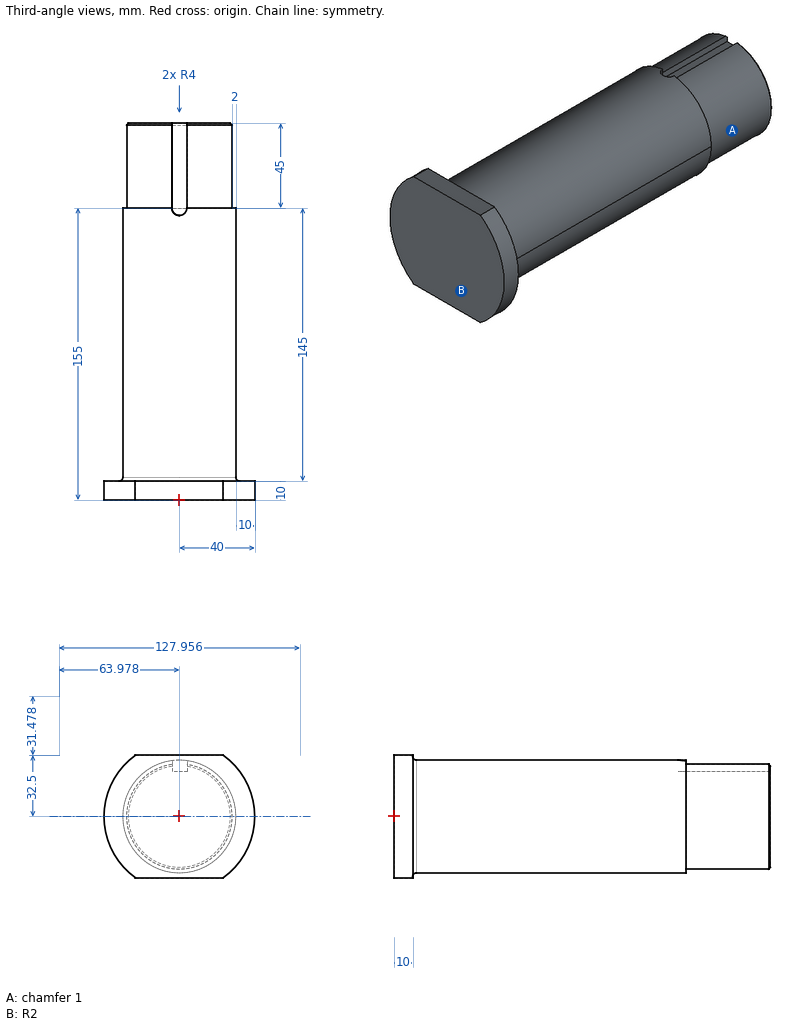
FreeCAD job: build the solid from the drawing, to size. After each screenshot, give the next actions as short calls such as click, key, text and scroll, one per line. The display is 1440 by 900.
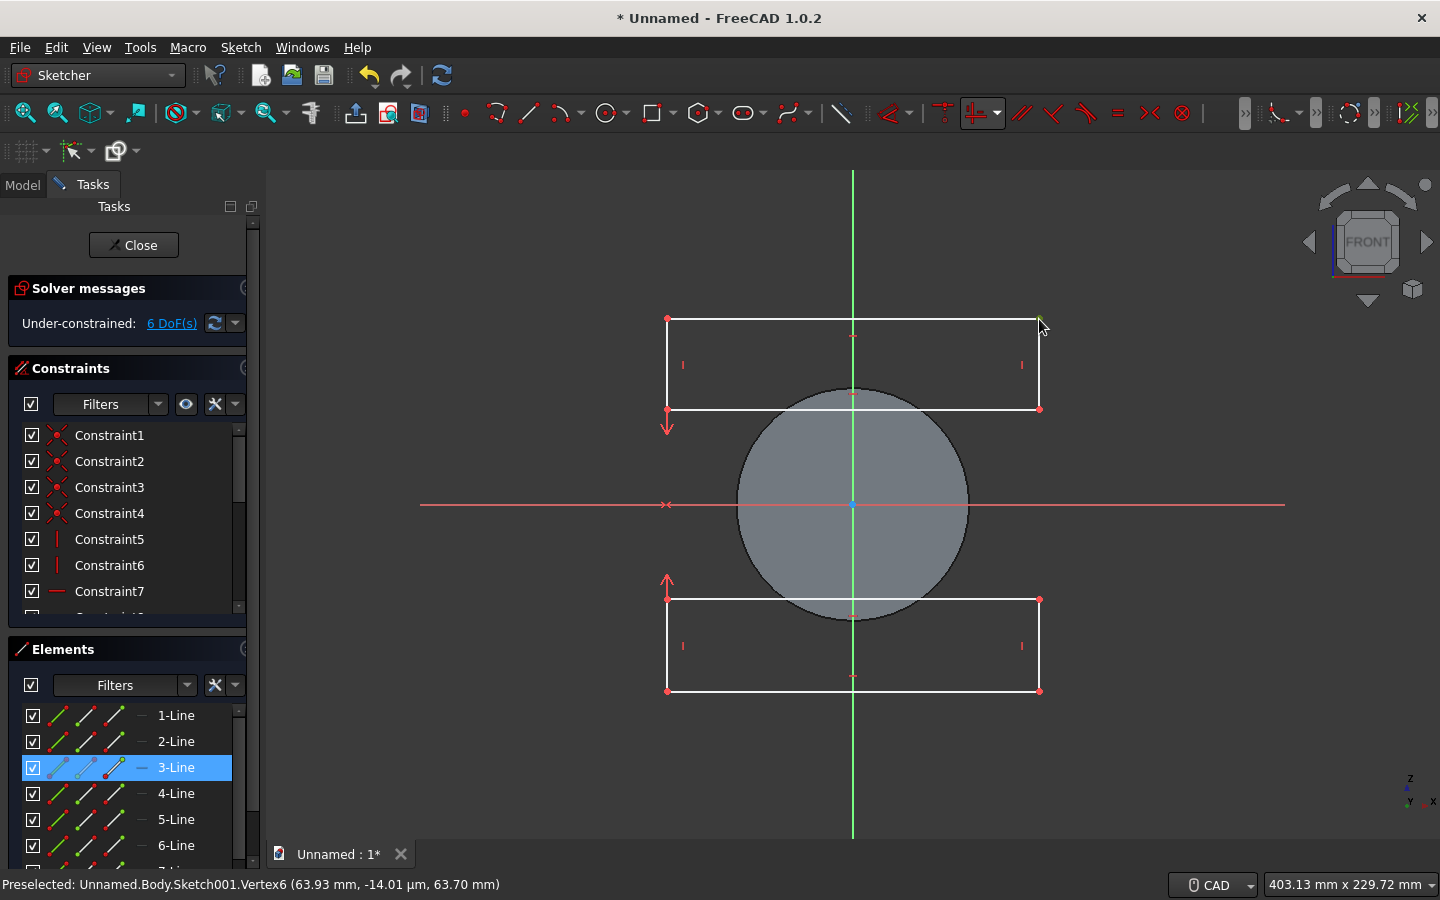
click(1039, 692)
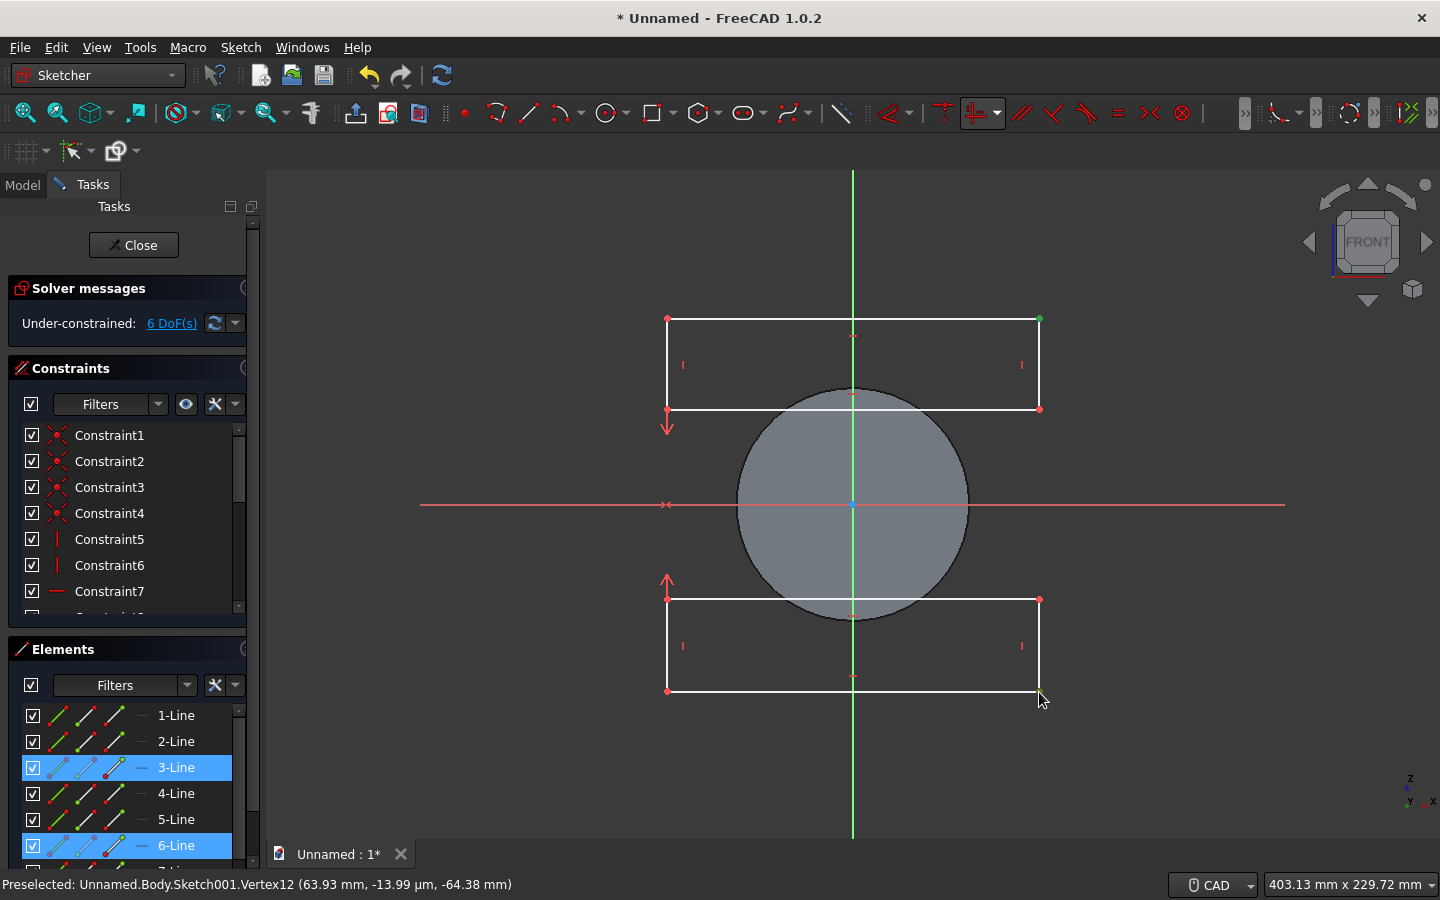
click(434, 505)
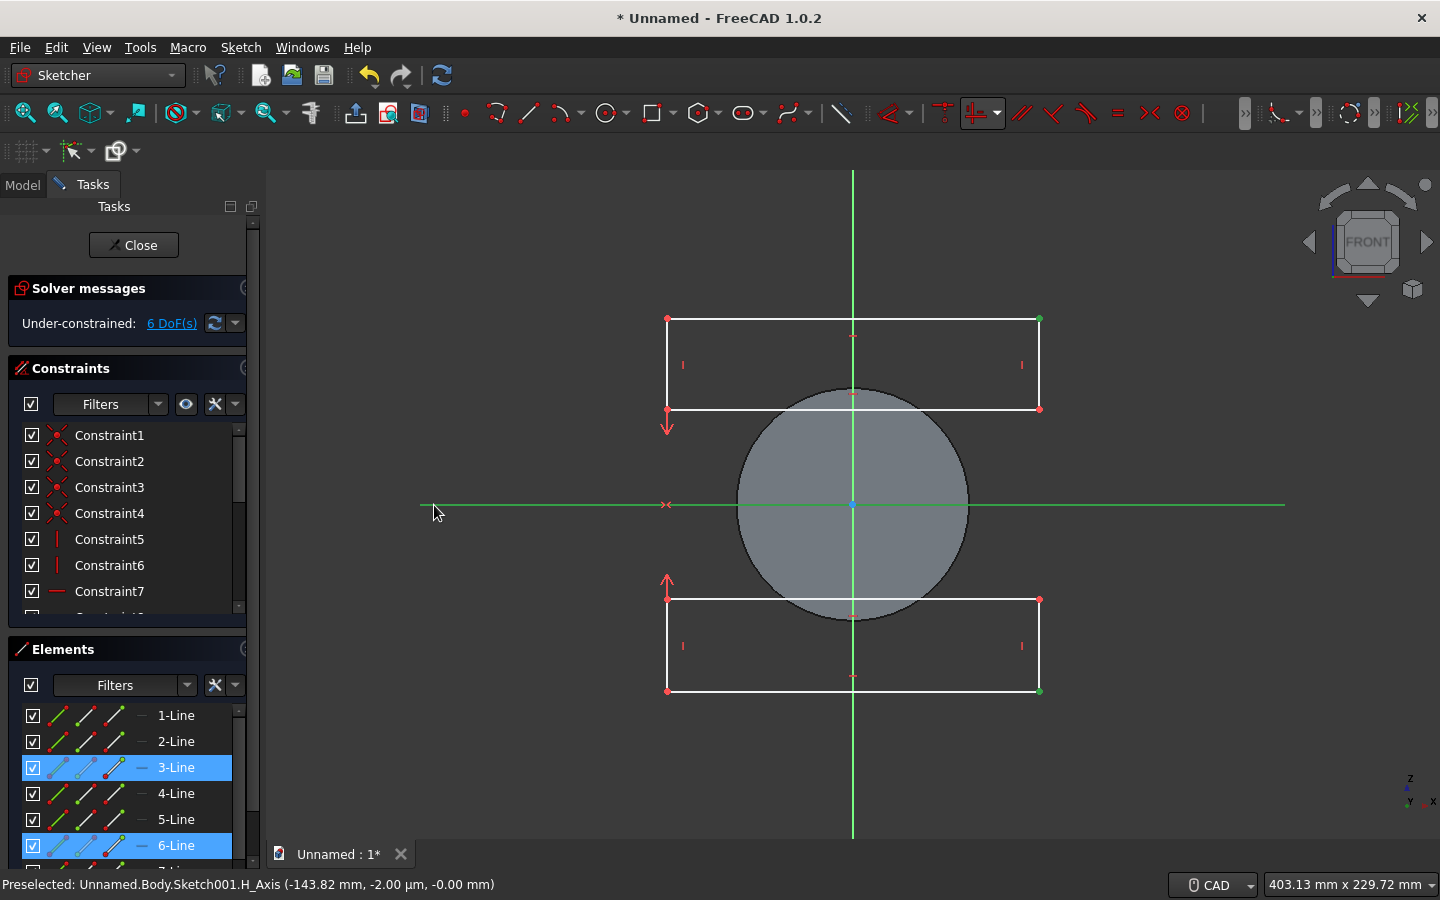
click(1150, 114)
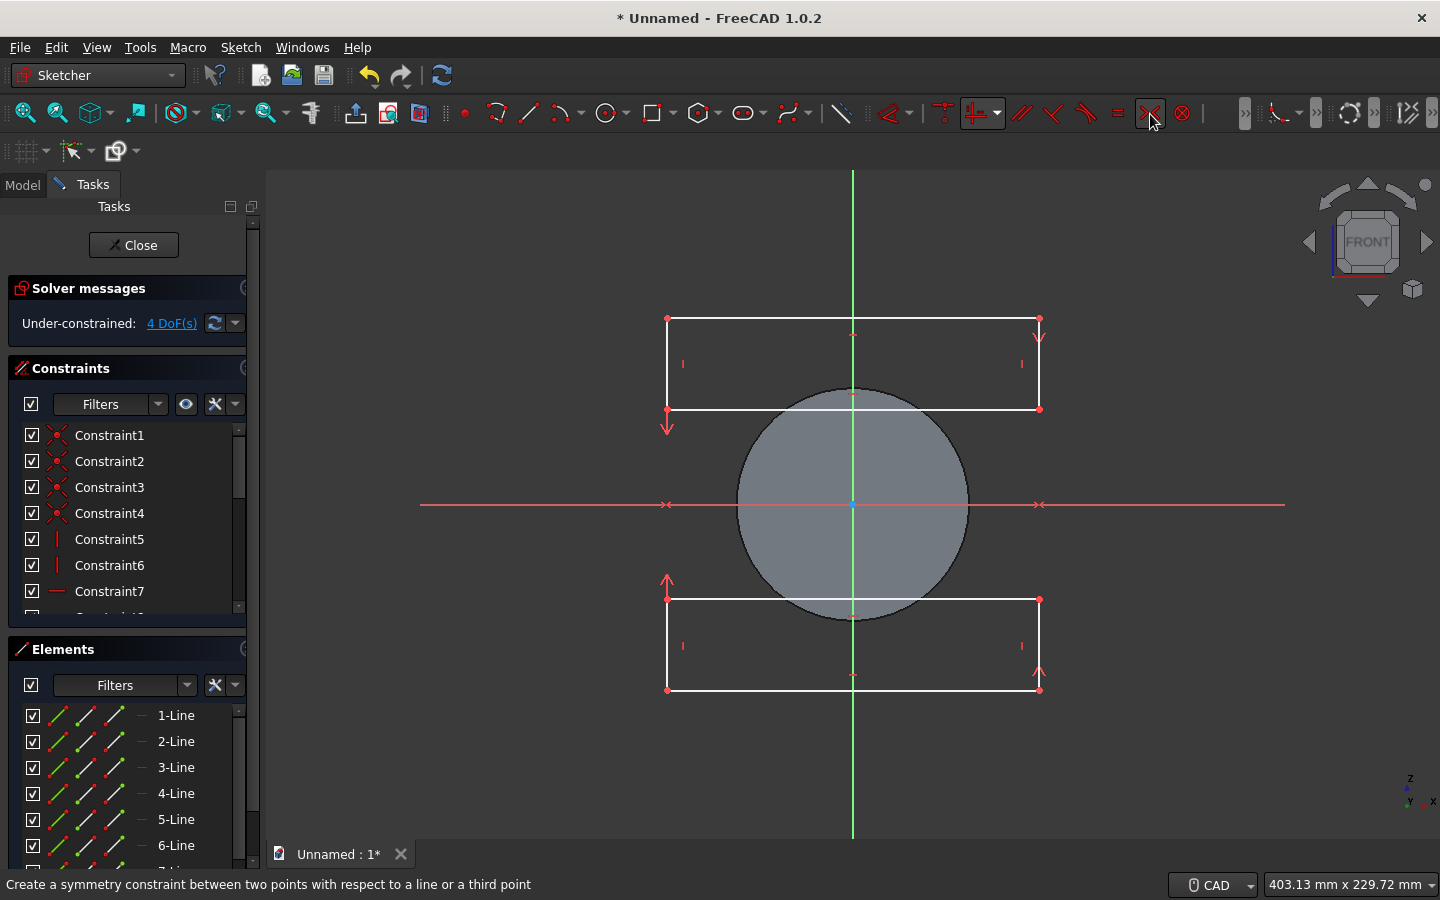
click(888, 114)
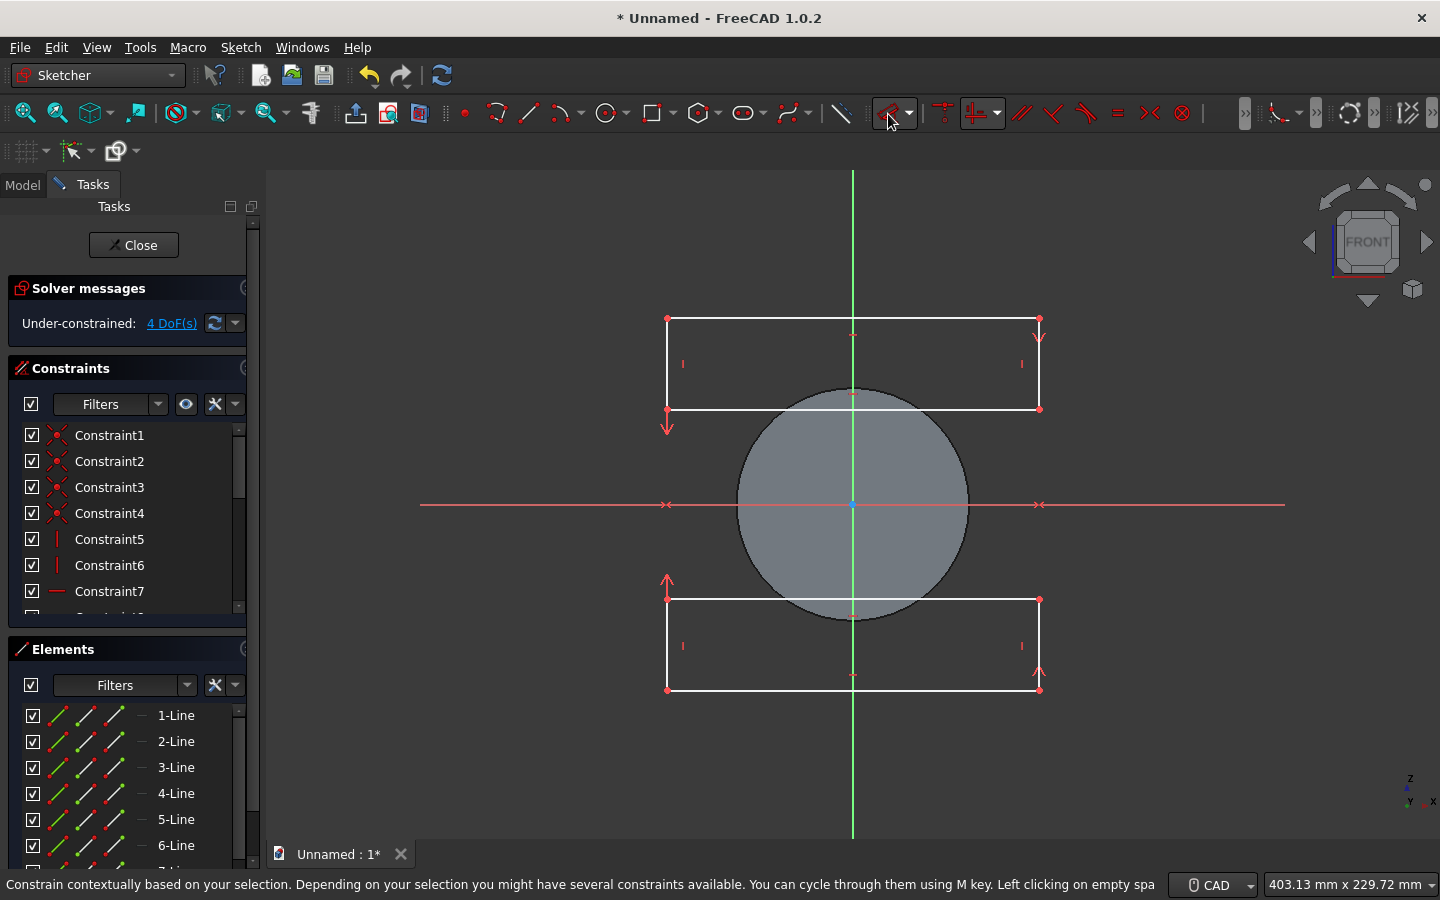
click(667, 410)
click(633, 457)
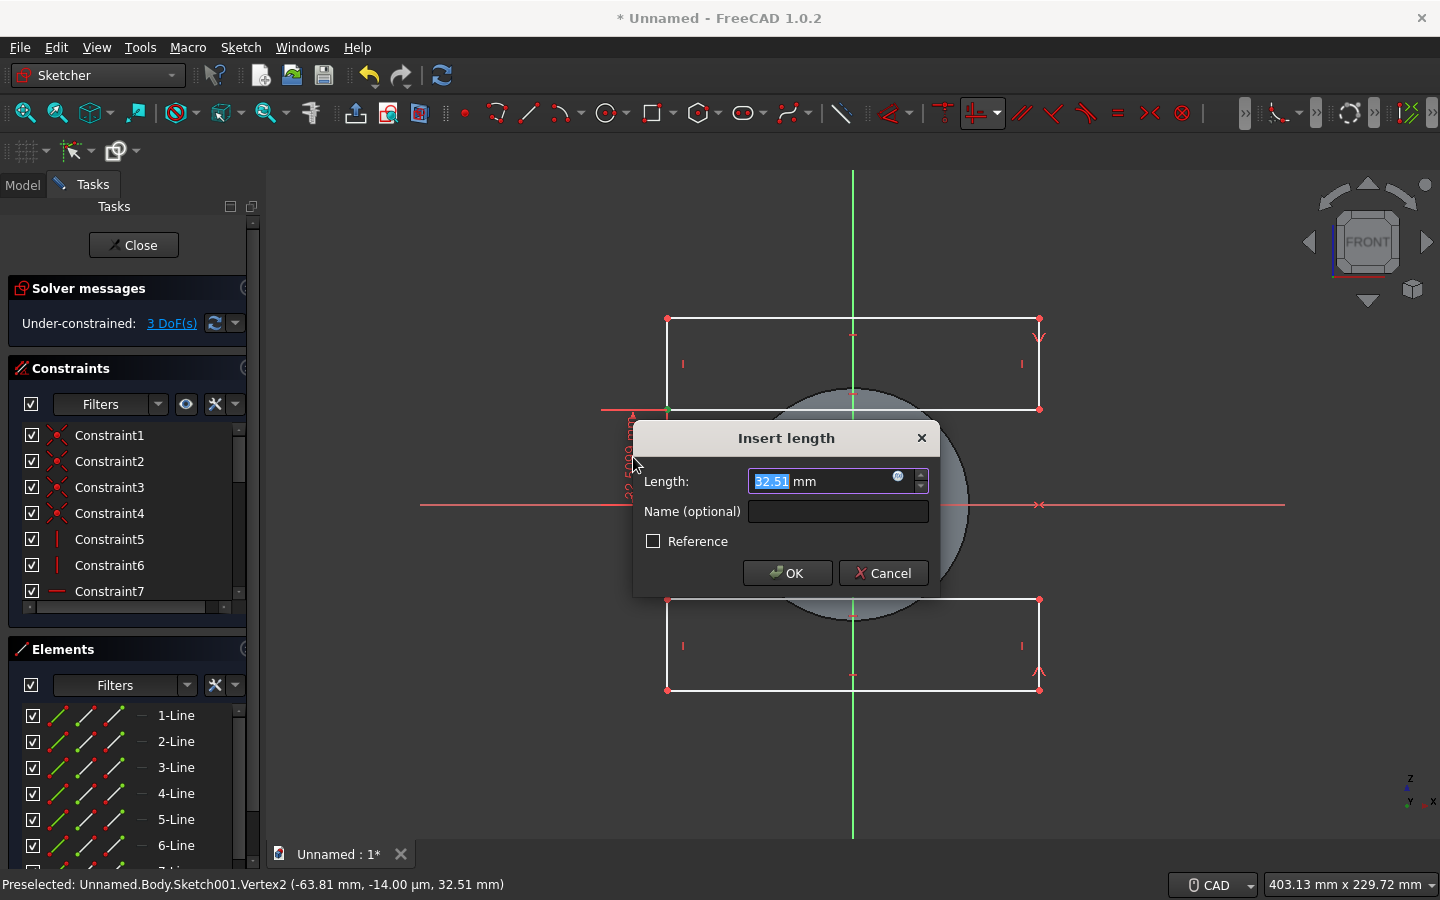
text(32.5)
key(Return)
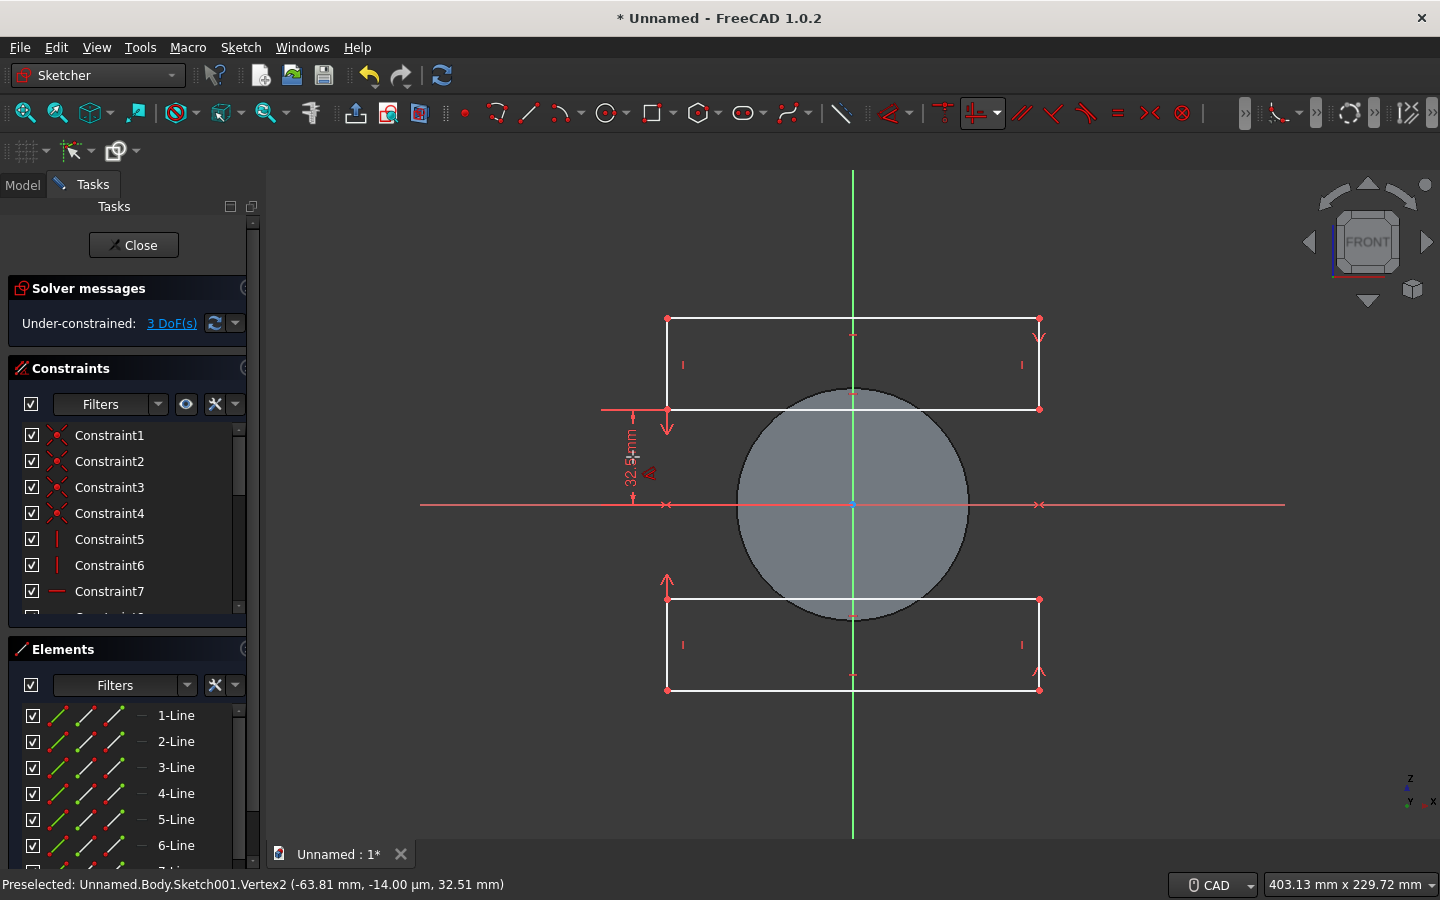
click(667, 346)
click(633, 364)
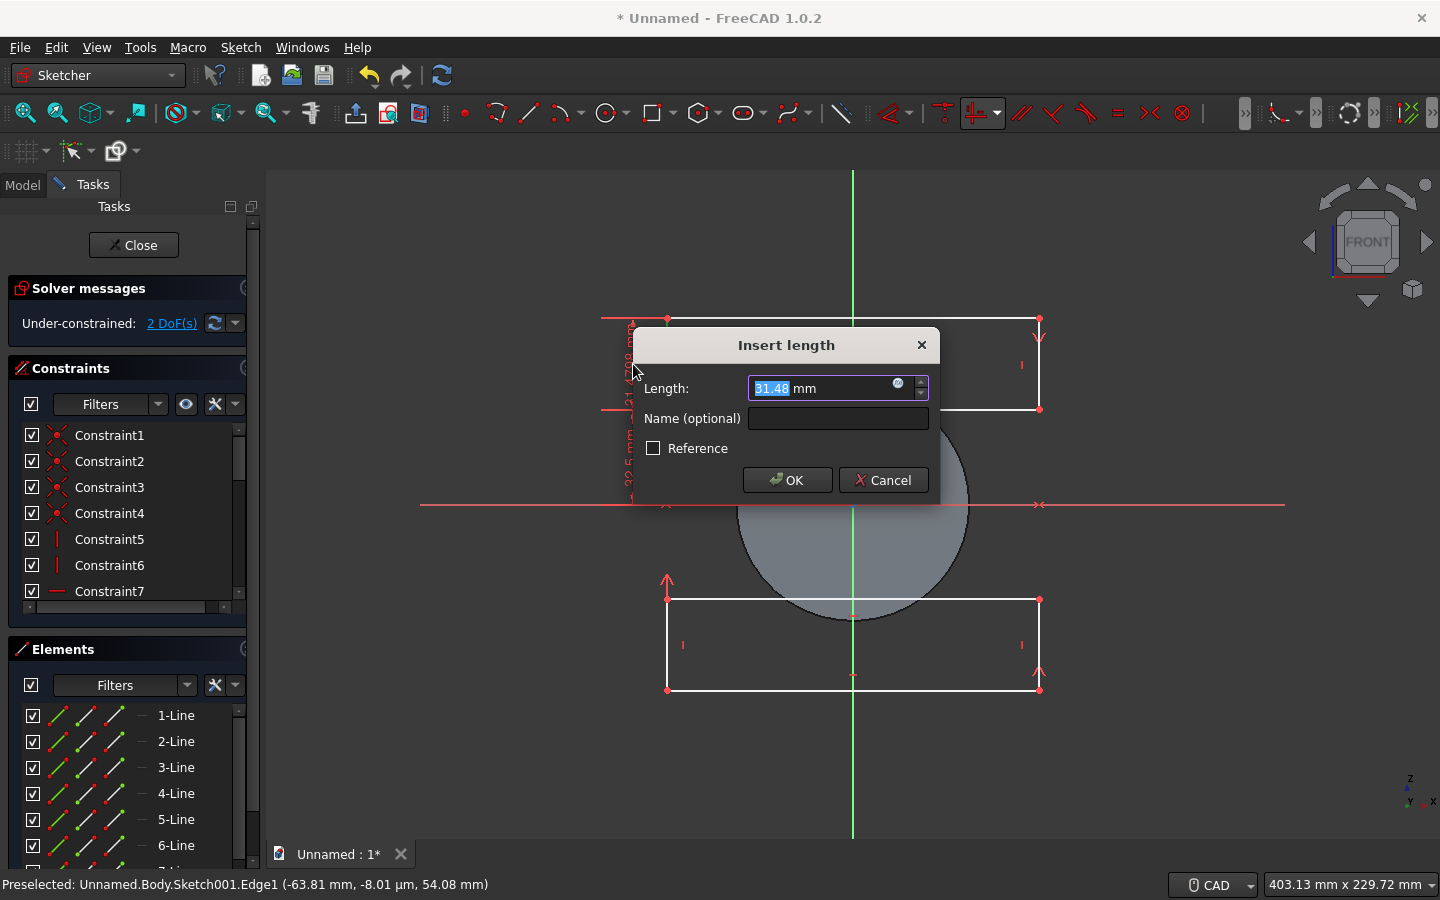
text(31.478)
key(Return)